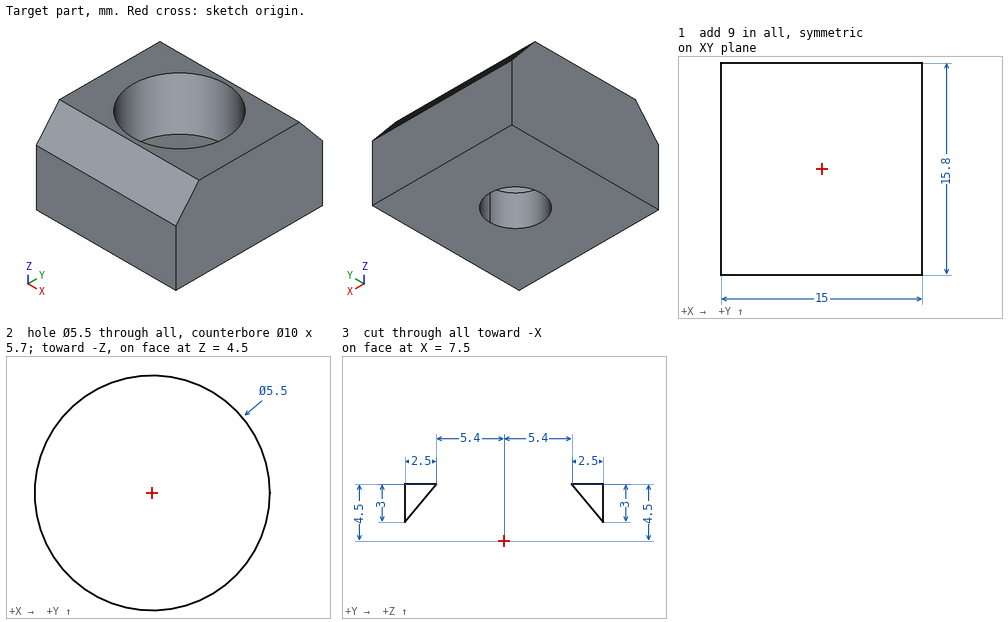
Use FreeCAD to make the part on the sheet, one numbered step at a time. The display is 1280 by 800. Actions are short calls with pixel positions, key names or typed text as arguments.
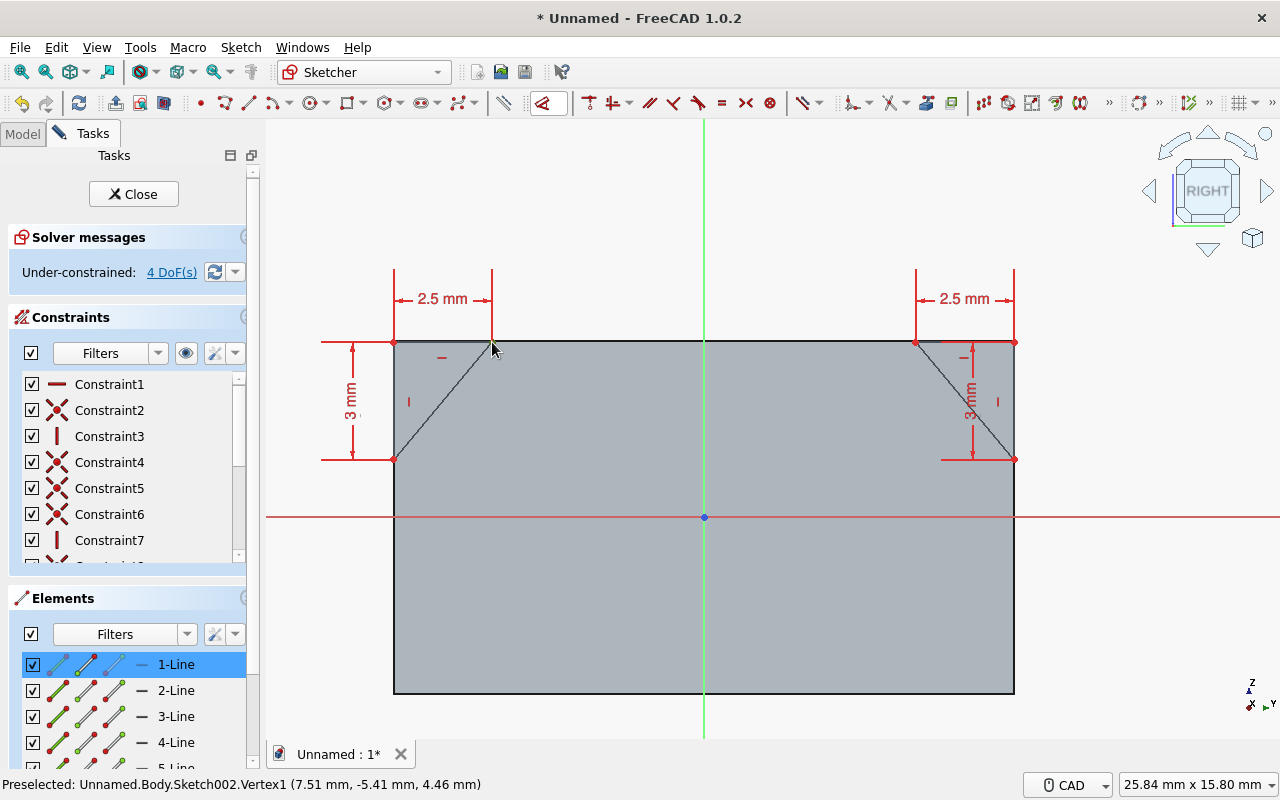
key(l)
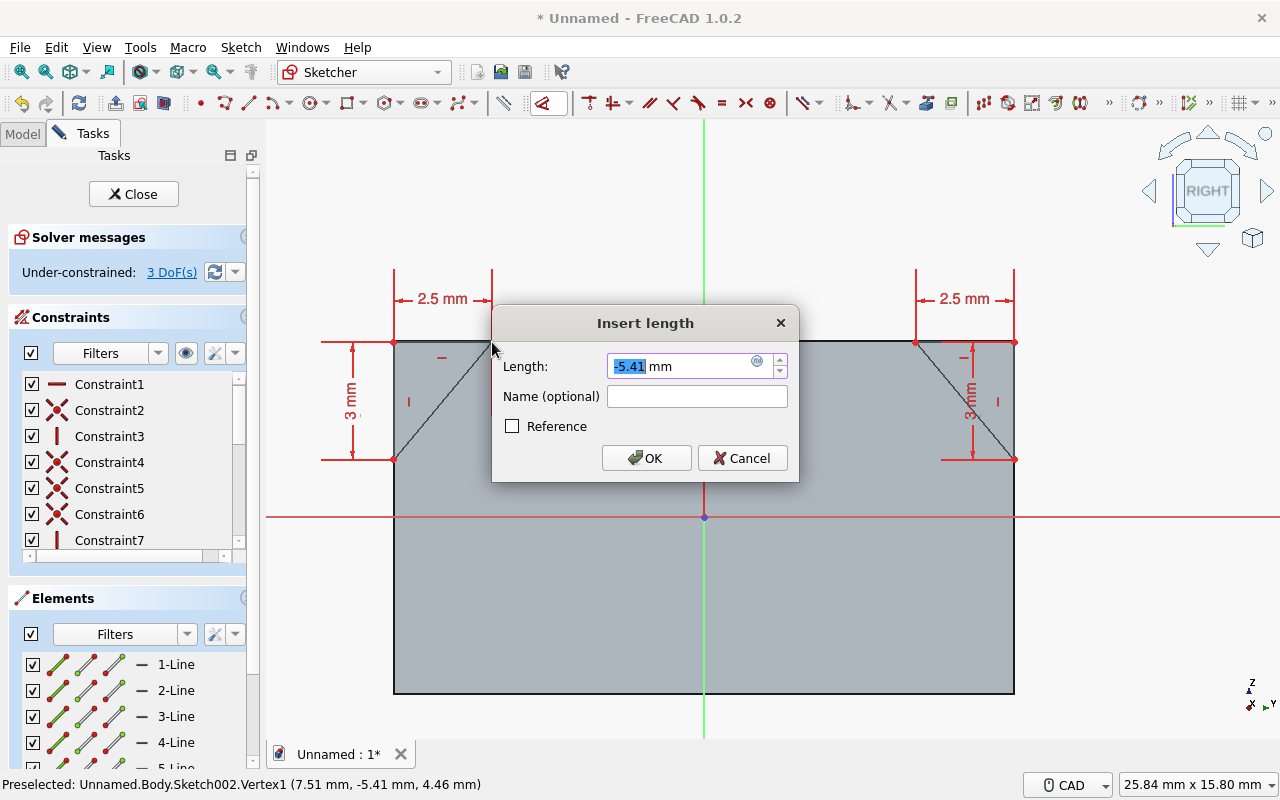
text(-5.4)
key(Return)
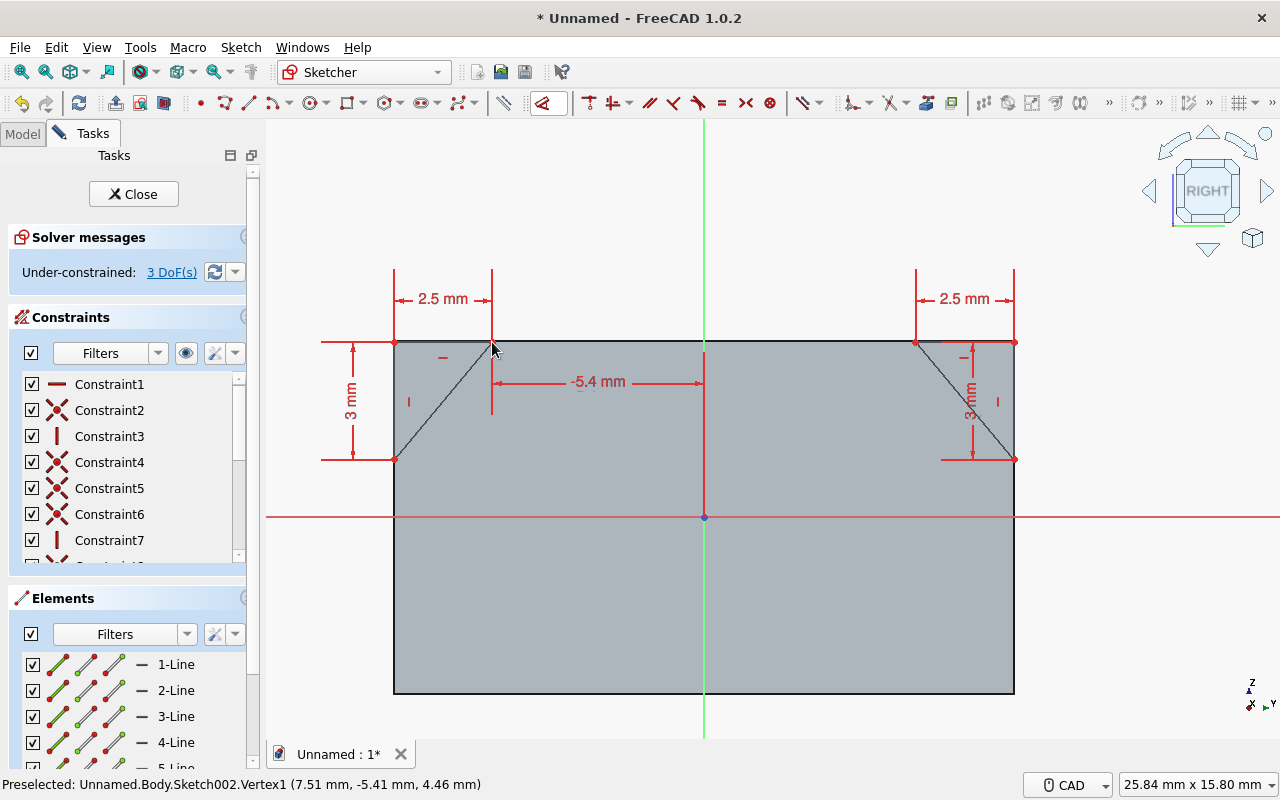
click(492, 342)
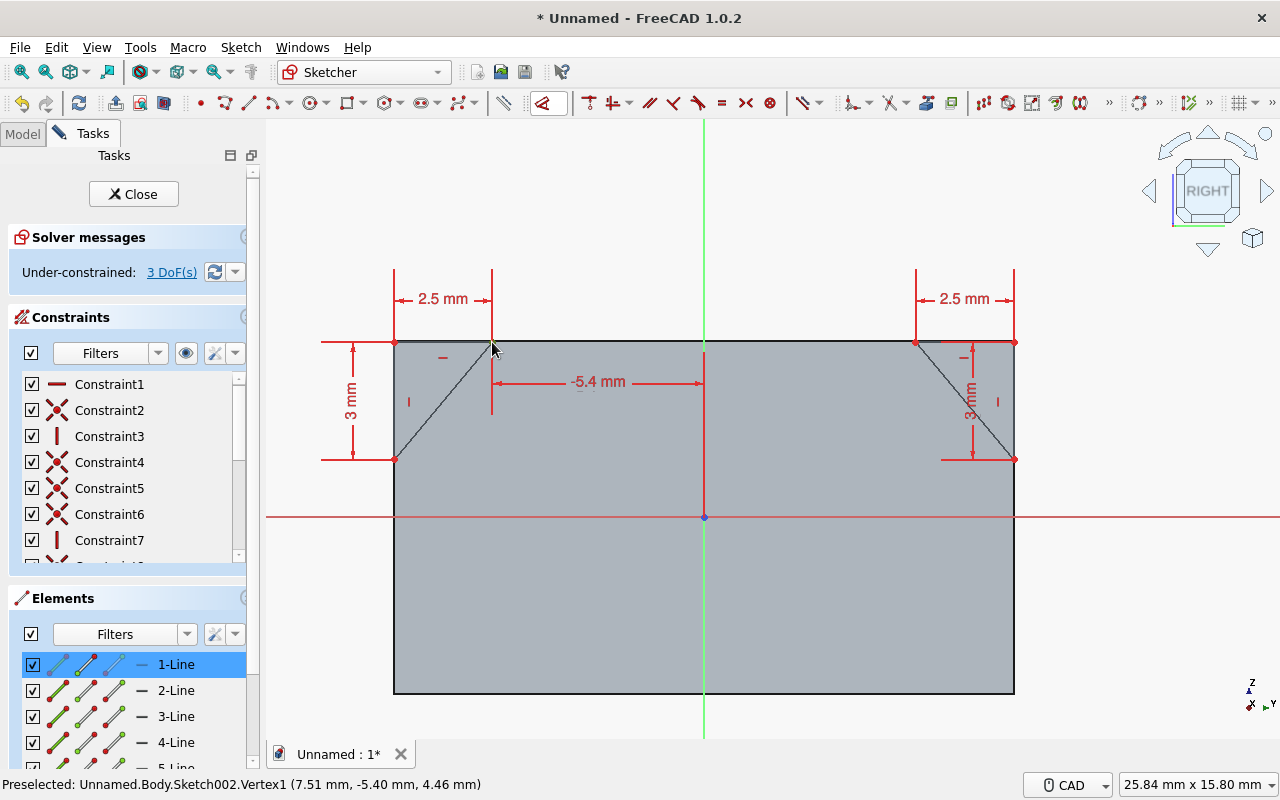
click(562, 104)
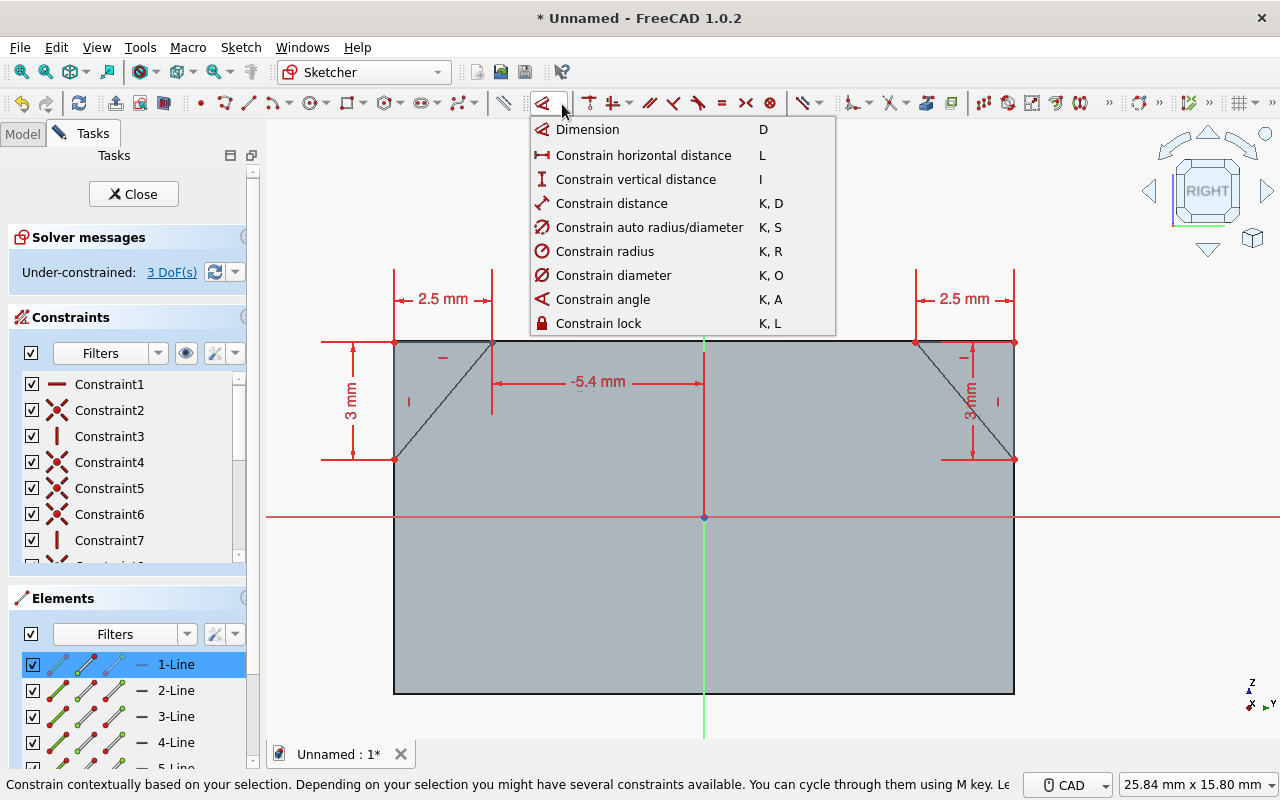
click(683, 179)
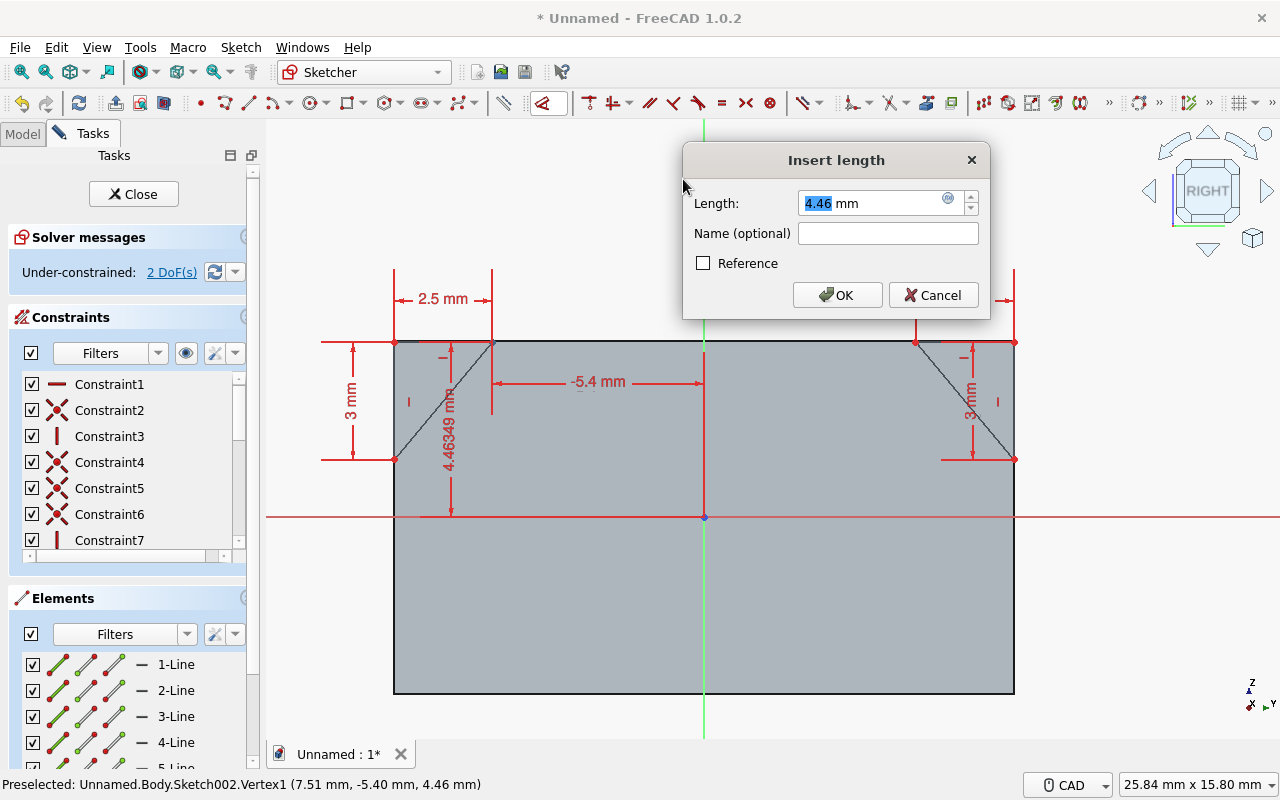
text(4.5)
key(Return)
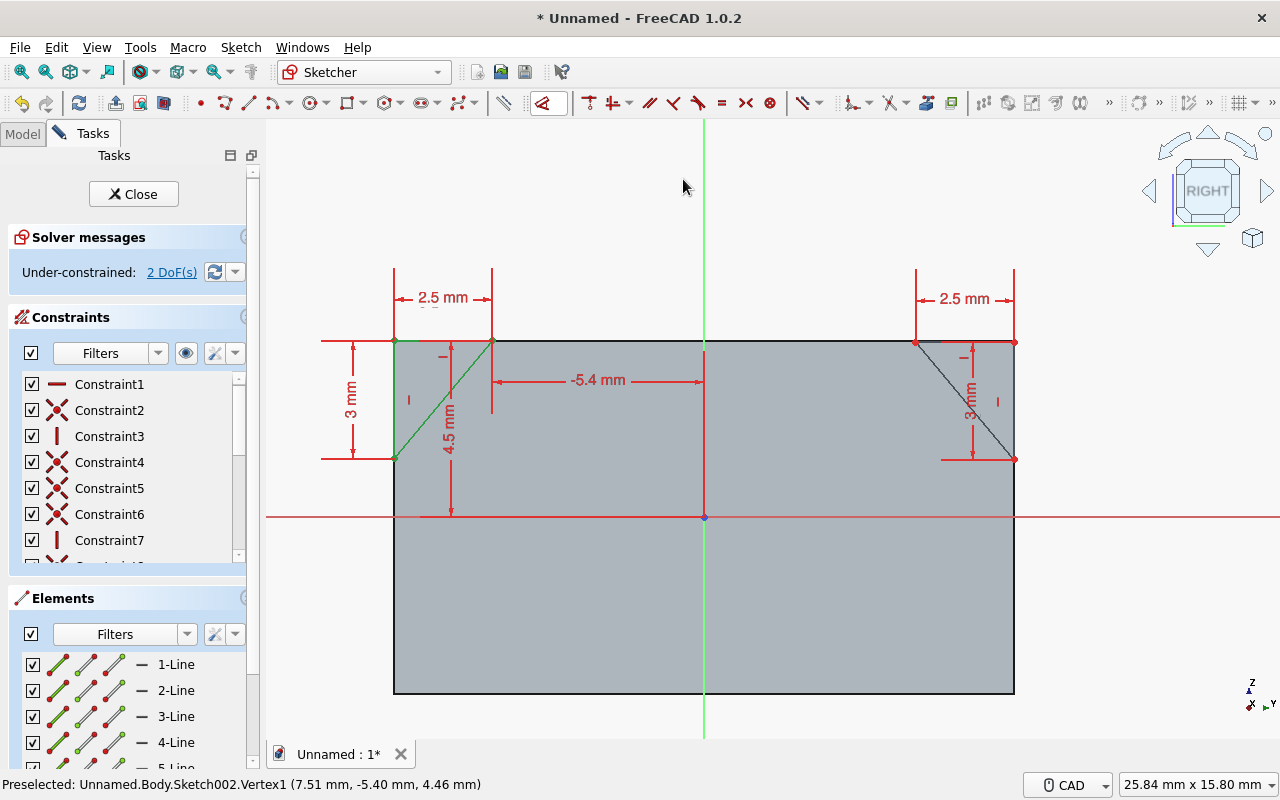
click(916, 342)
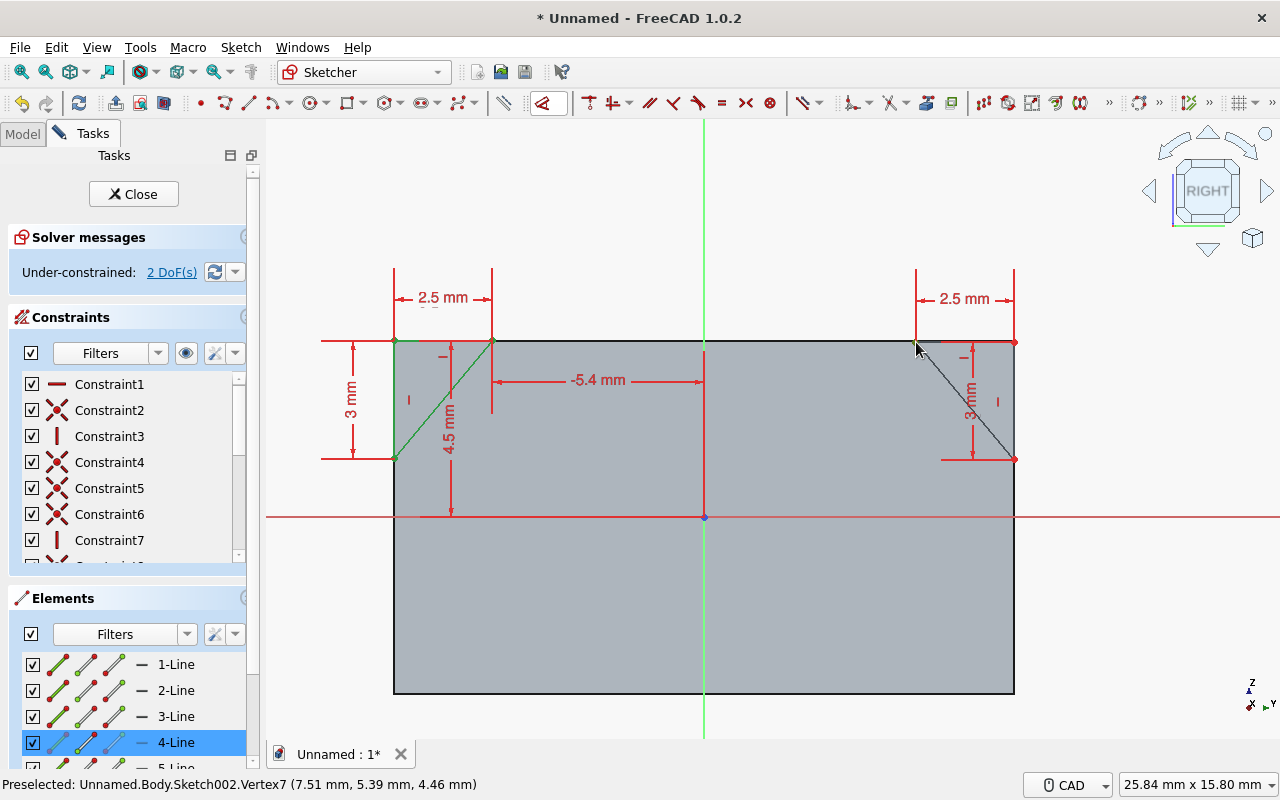
key(l)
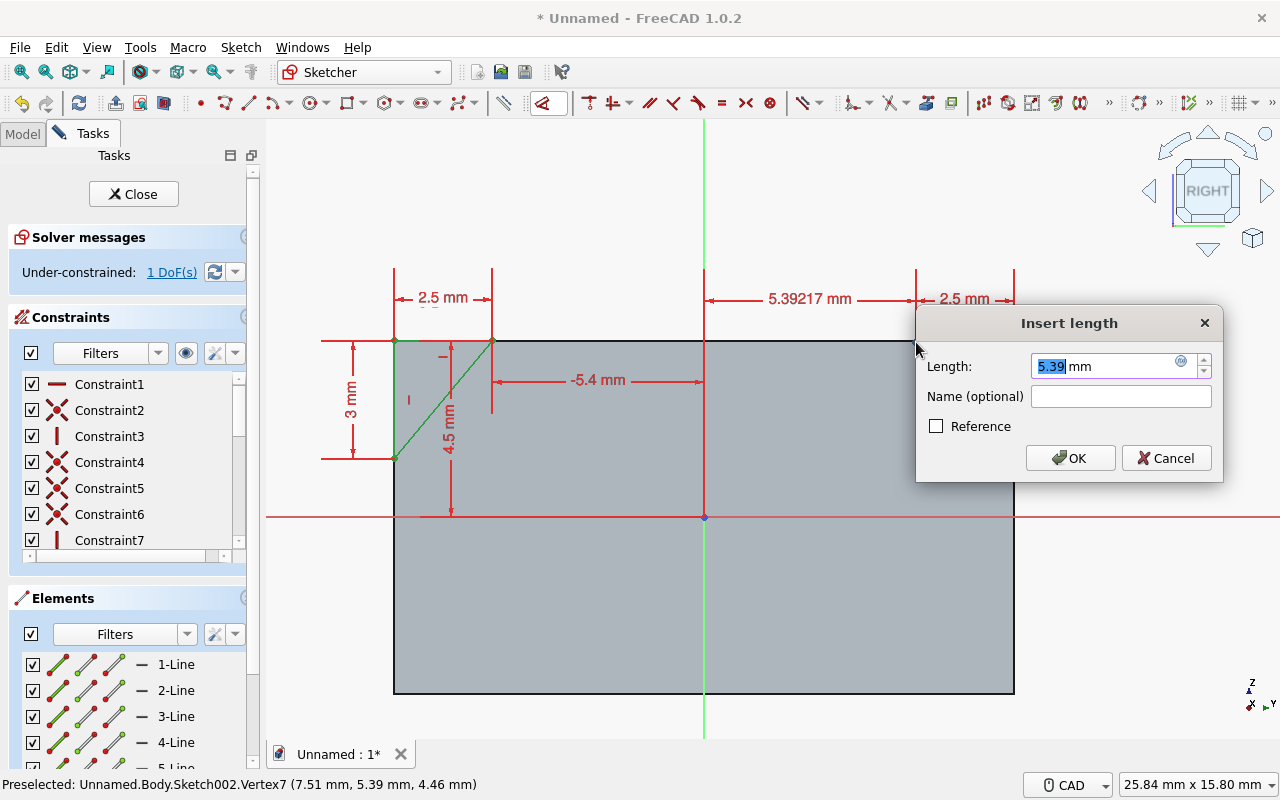
text(5.4)
key(Return)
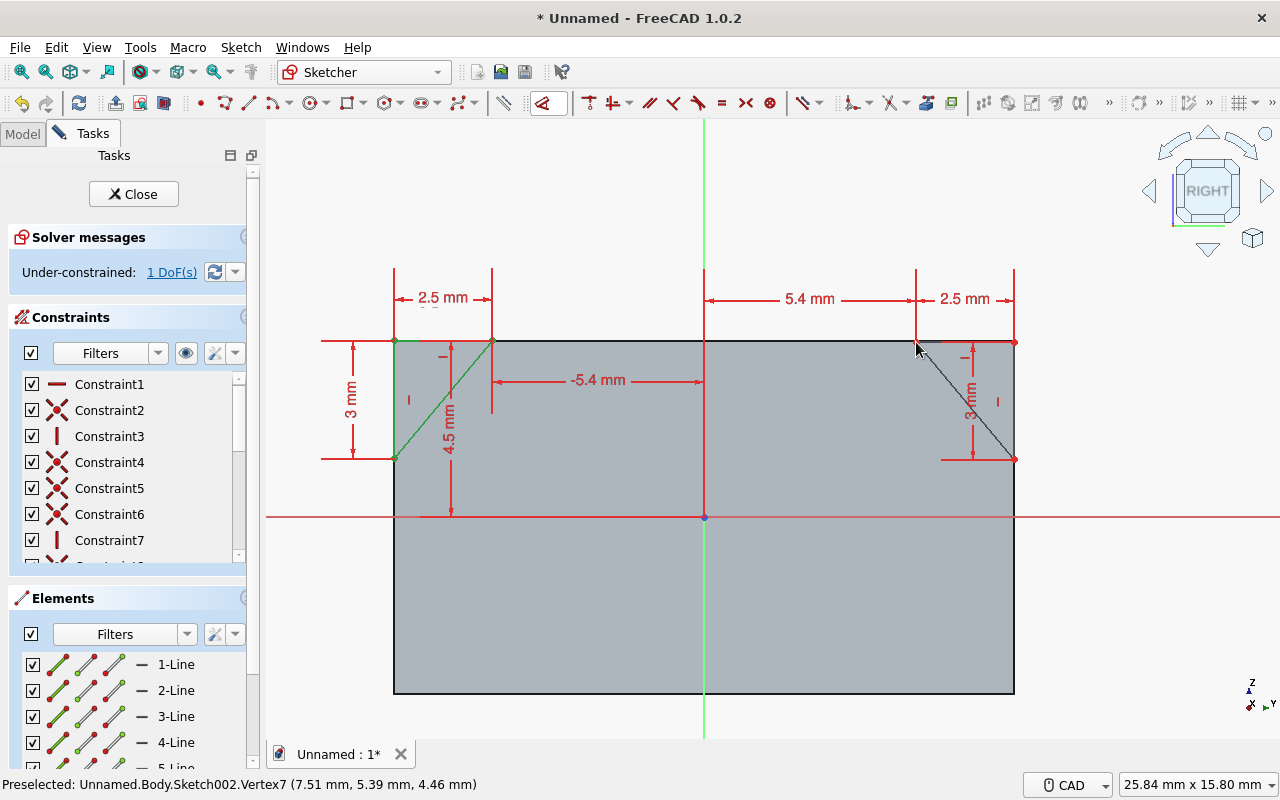
click(916, 342)